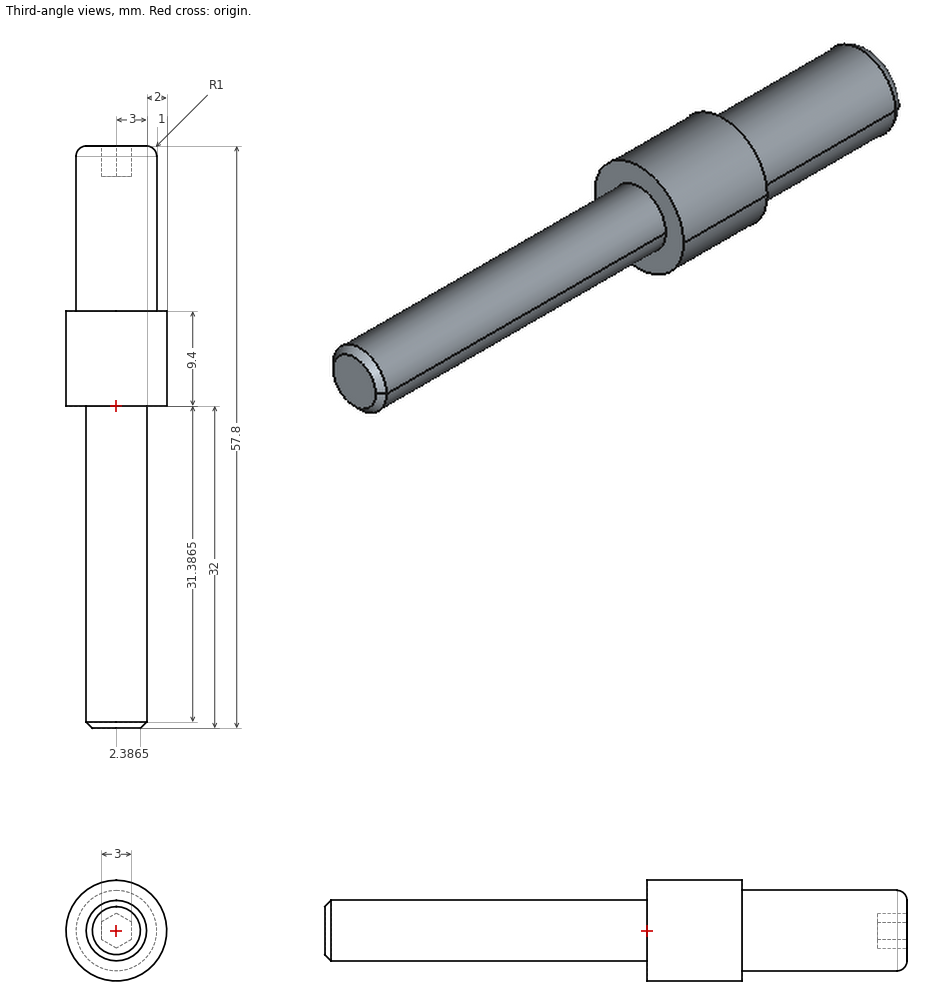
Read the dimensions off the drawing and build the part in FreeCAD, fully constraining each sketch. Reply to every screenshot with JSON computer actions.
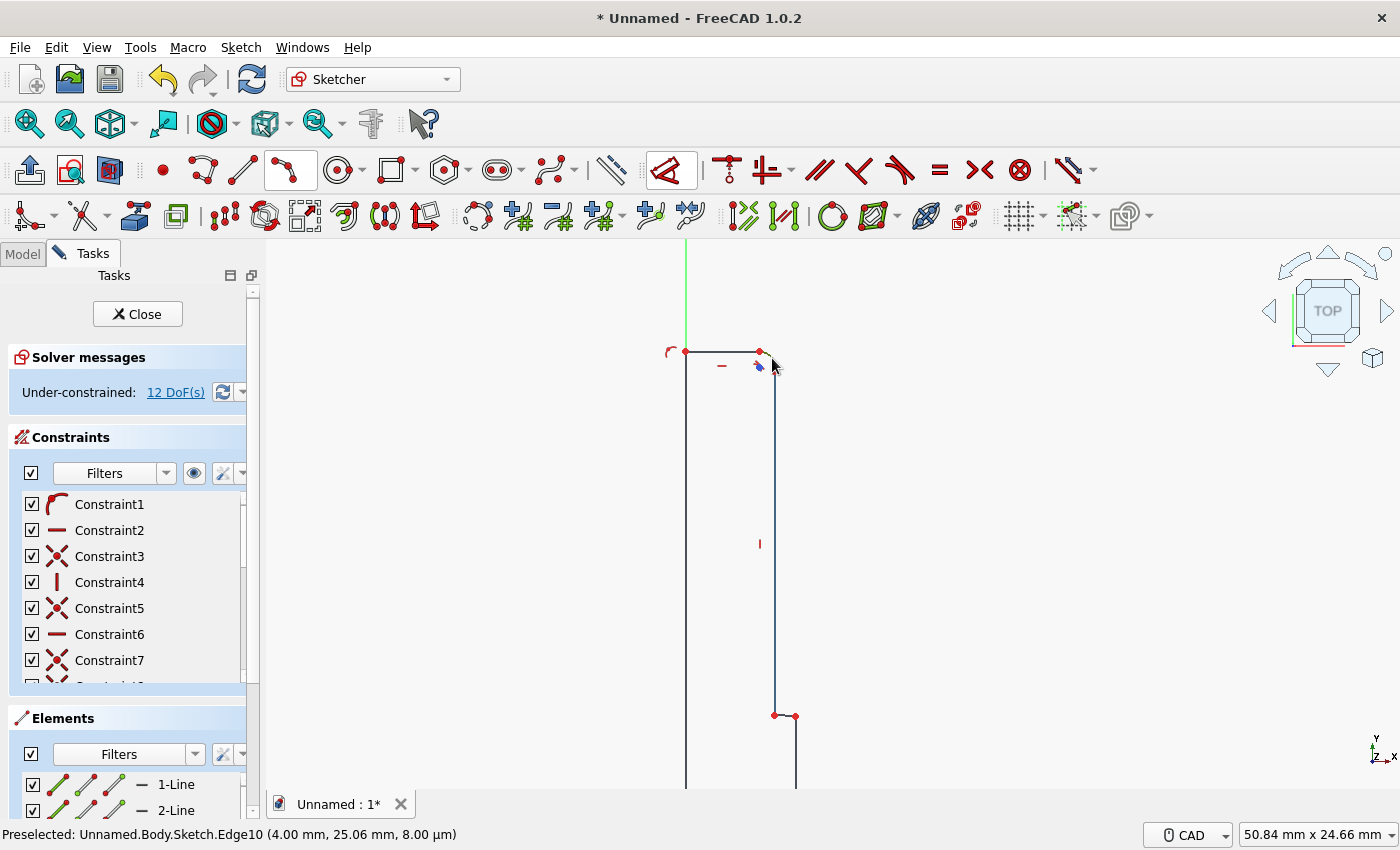
{"action": "left_click", "coordinate": [900, 170]}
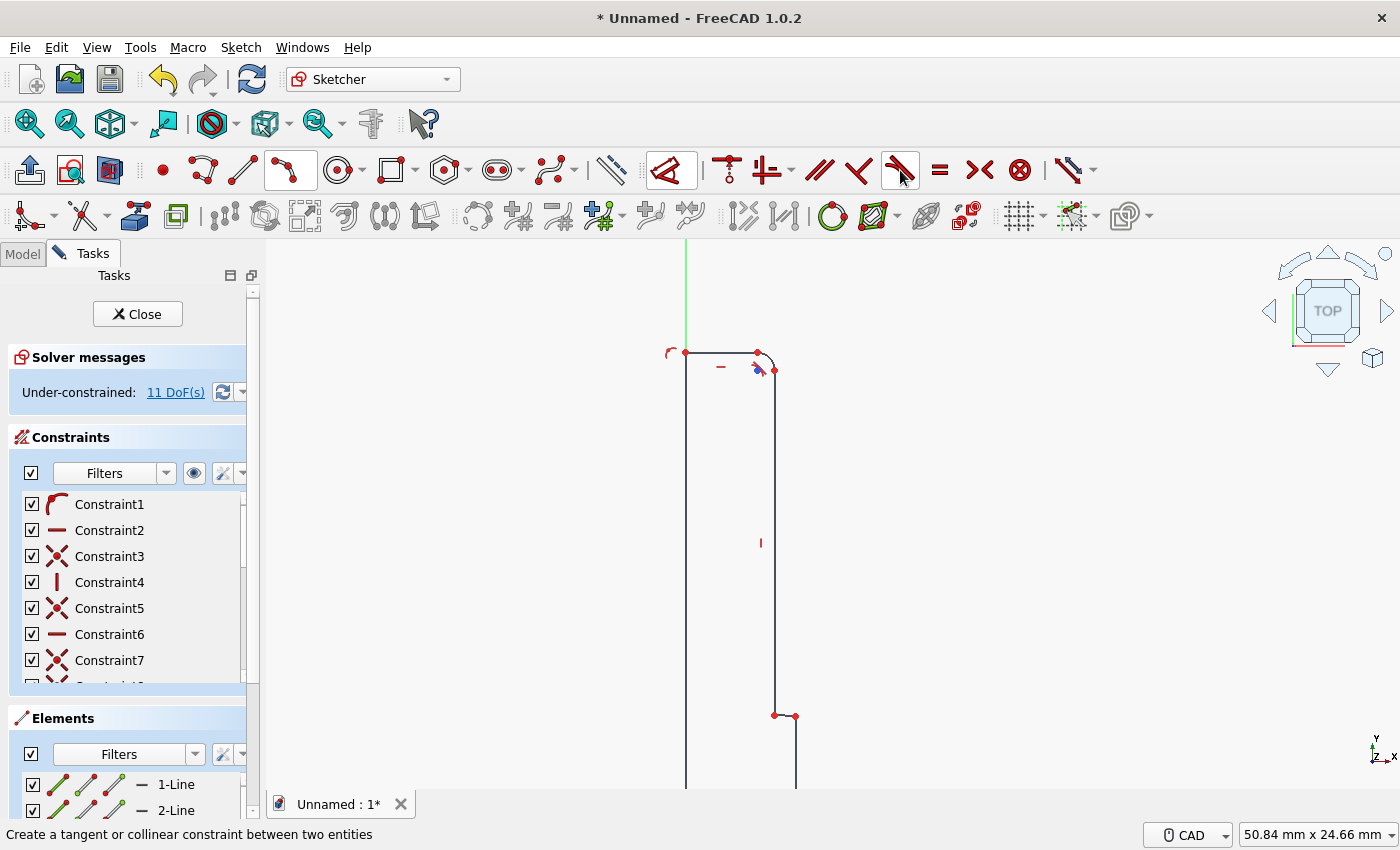
{"action": "scroll", "coordinate": [772, 358], "scroll_direction": "down", "scroll_amount": 7}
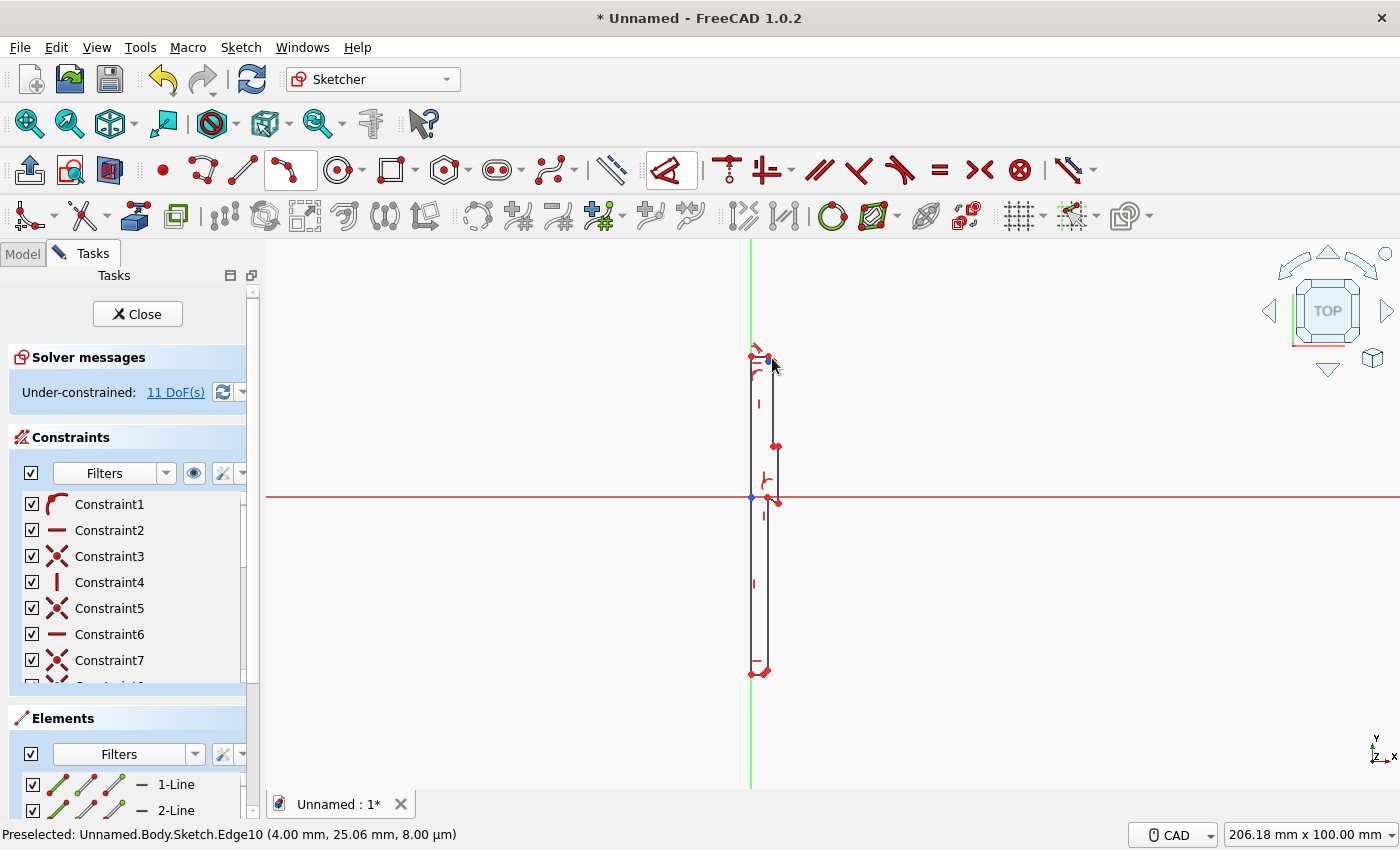
{"action": "scroll", "coordinate": [775, 502], "scroll_direction": "up", "scroll_amount": 8}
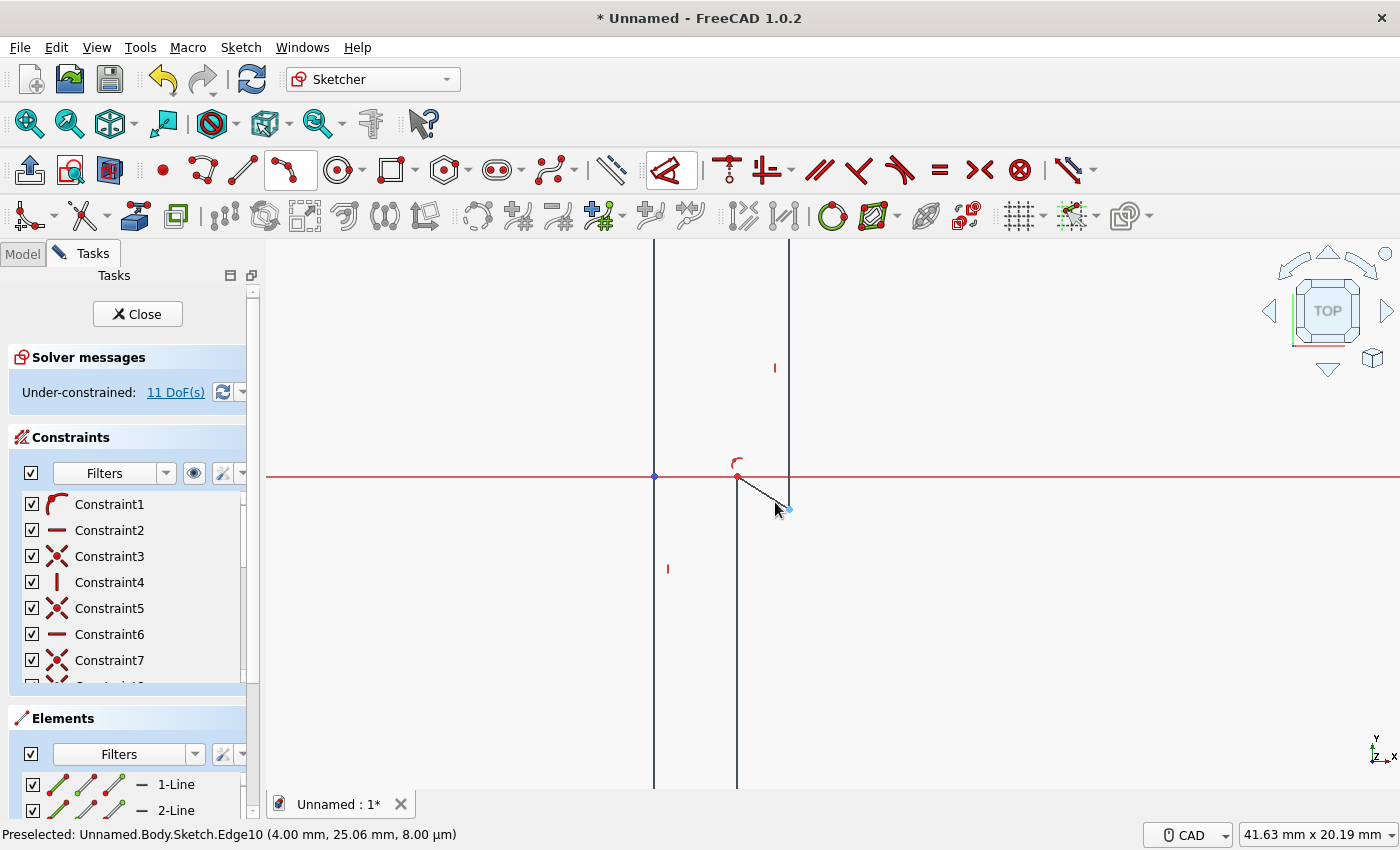
{"action": "left_click", "coordinate": [774, 500]}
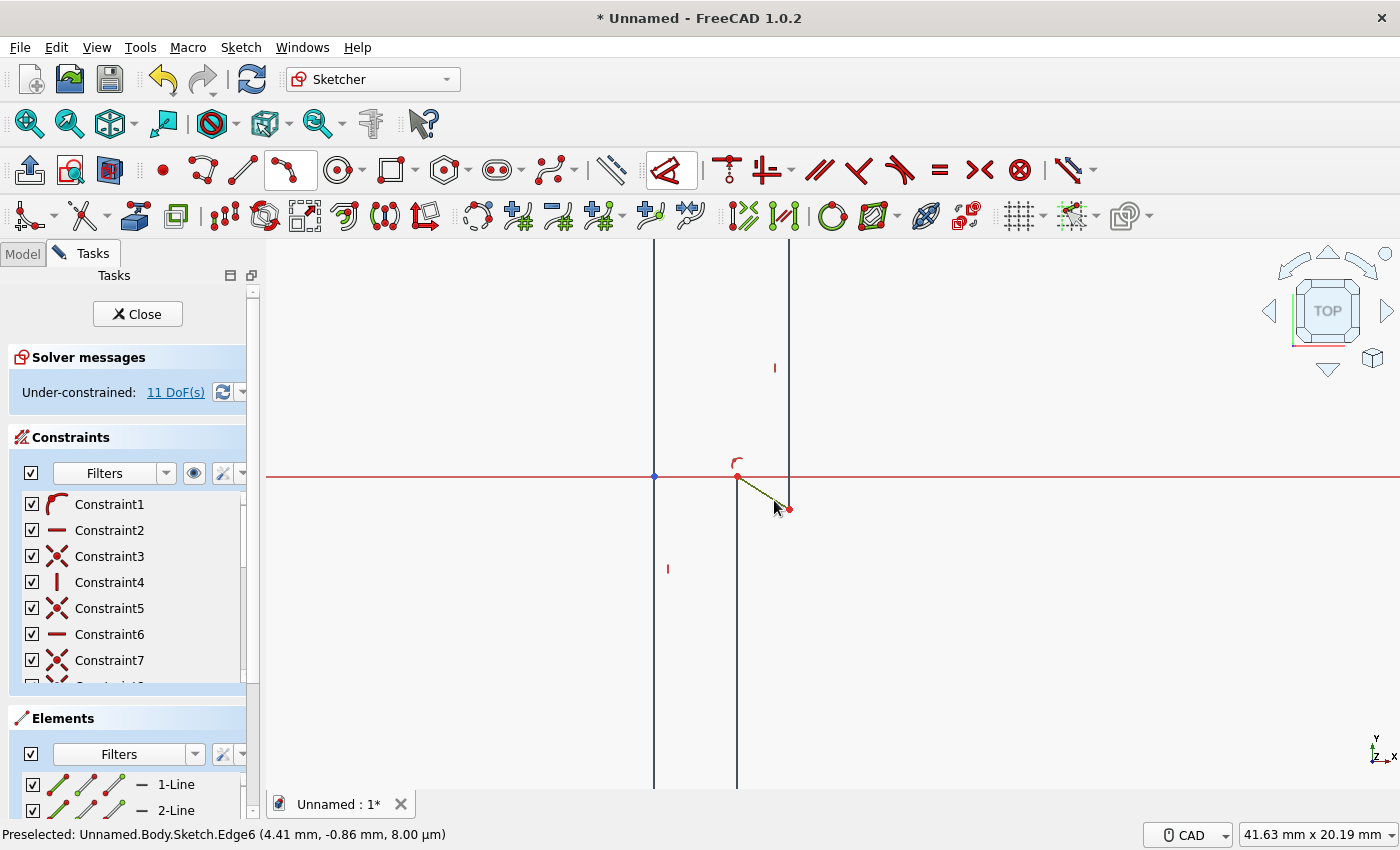
{"action": "left_click", "coordinate": [794, 170]}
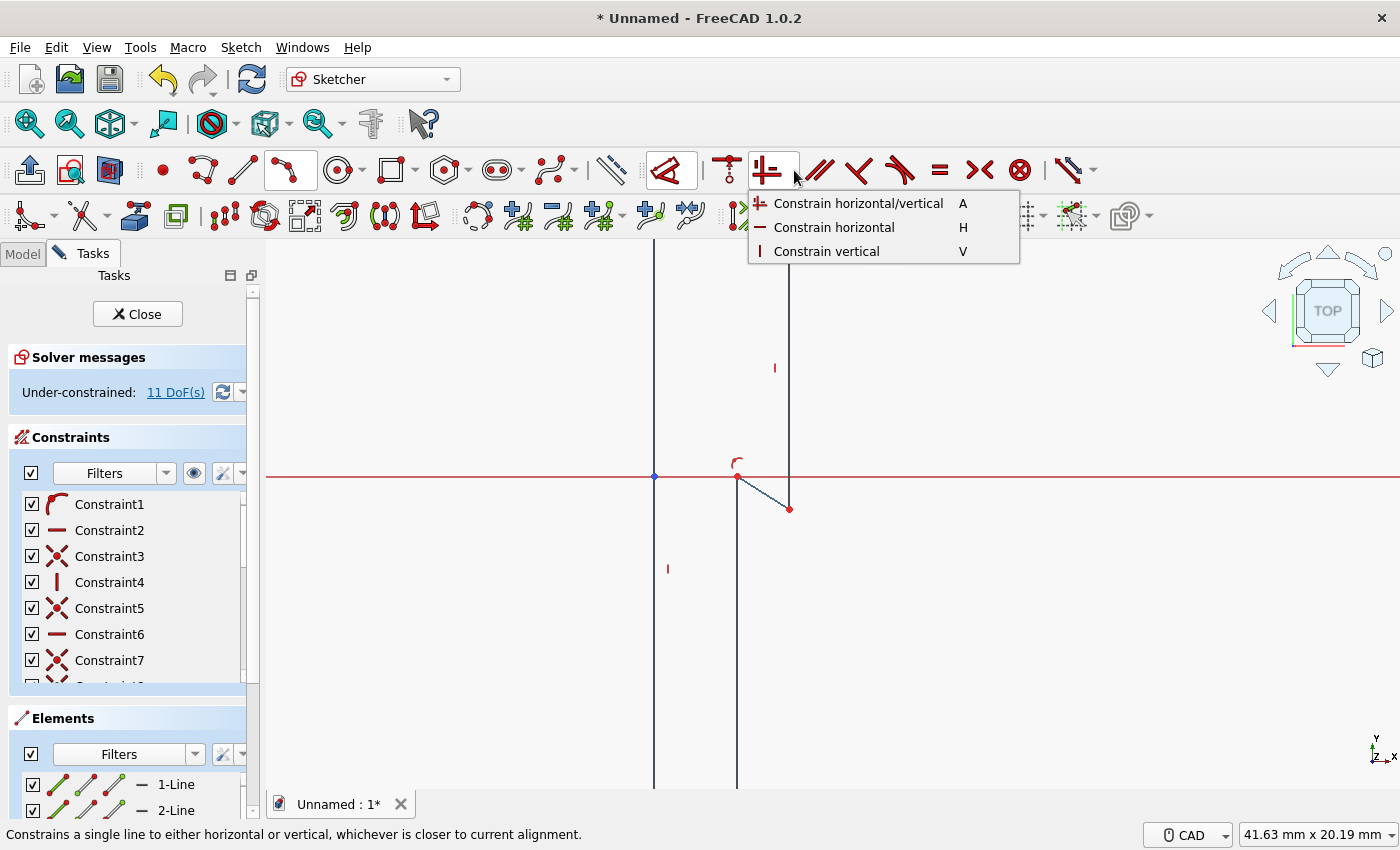
{"action": "left_click", "coordinate": [884, 227]}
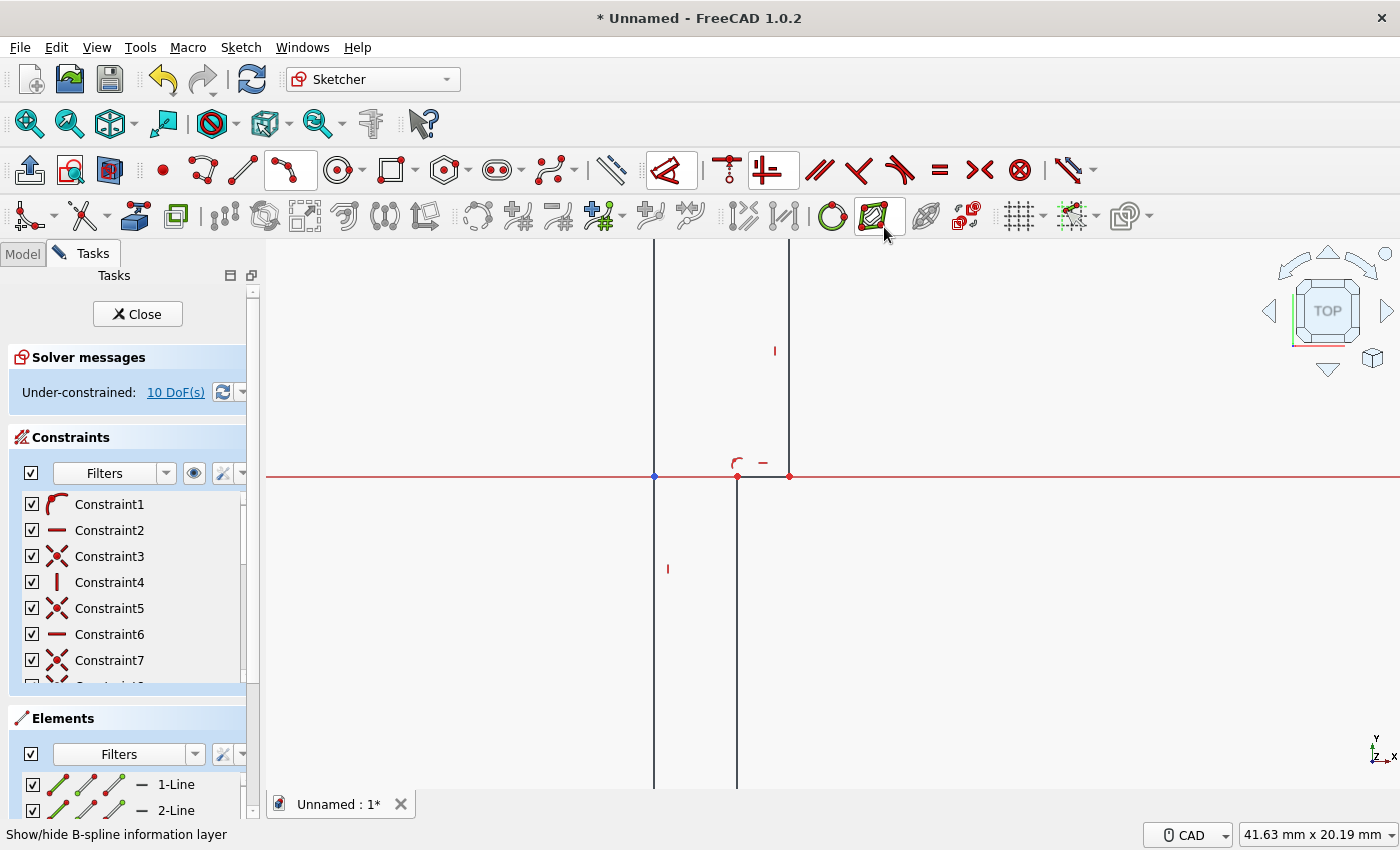
{"action": "scroll", "coordinate": [775, 502], "scroll_direction": "down", "scroll_amount": 8}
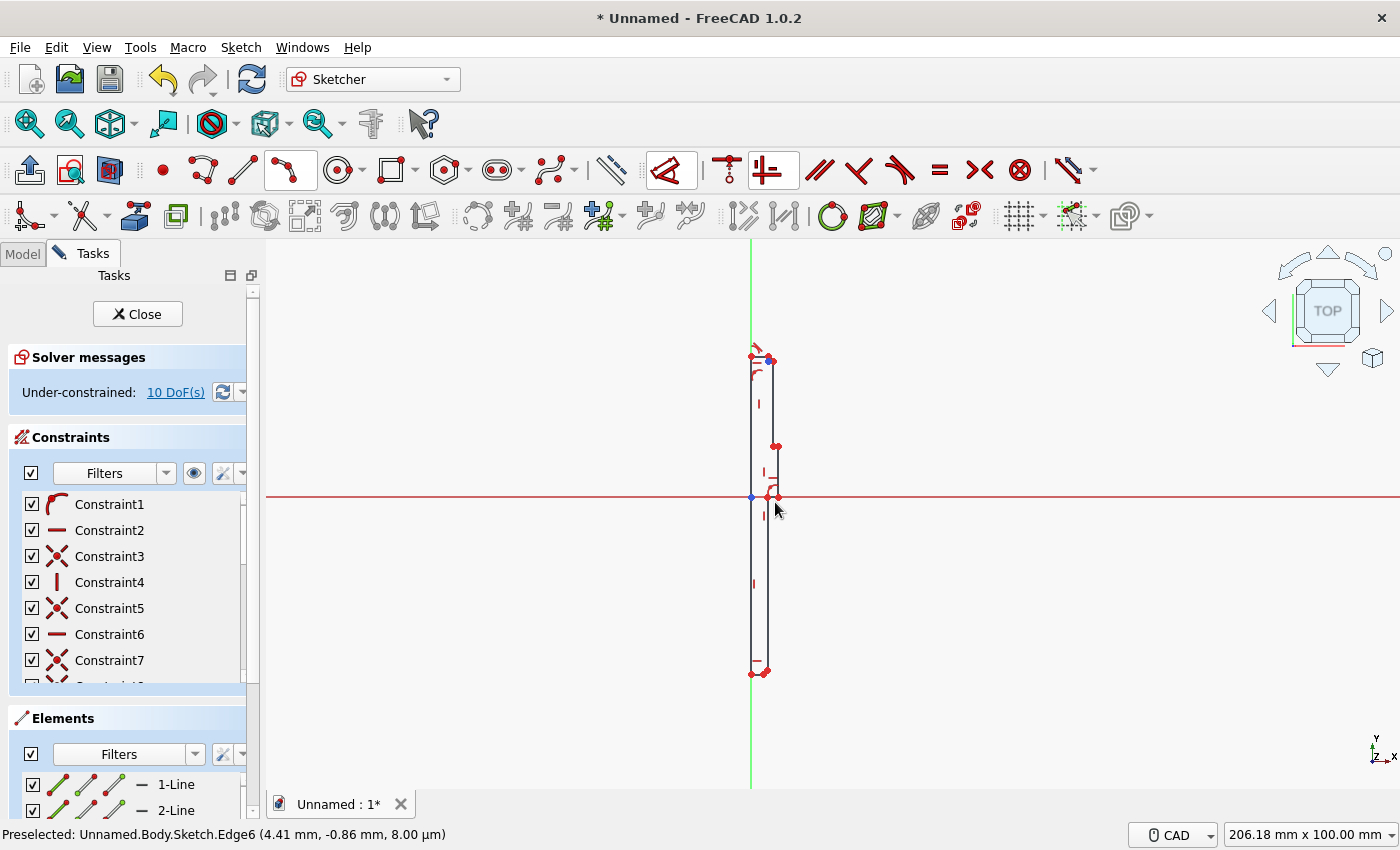
{"action": "scroll", "coordinate": [776, 446], "scroll_direction": "up", "scroll_amount": 10}